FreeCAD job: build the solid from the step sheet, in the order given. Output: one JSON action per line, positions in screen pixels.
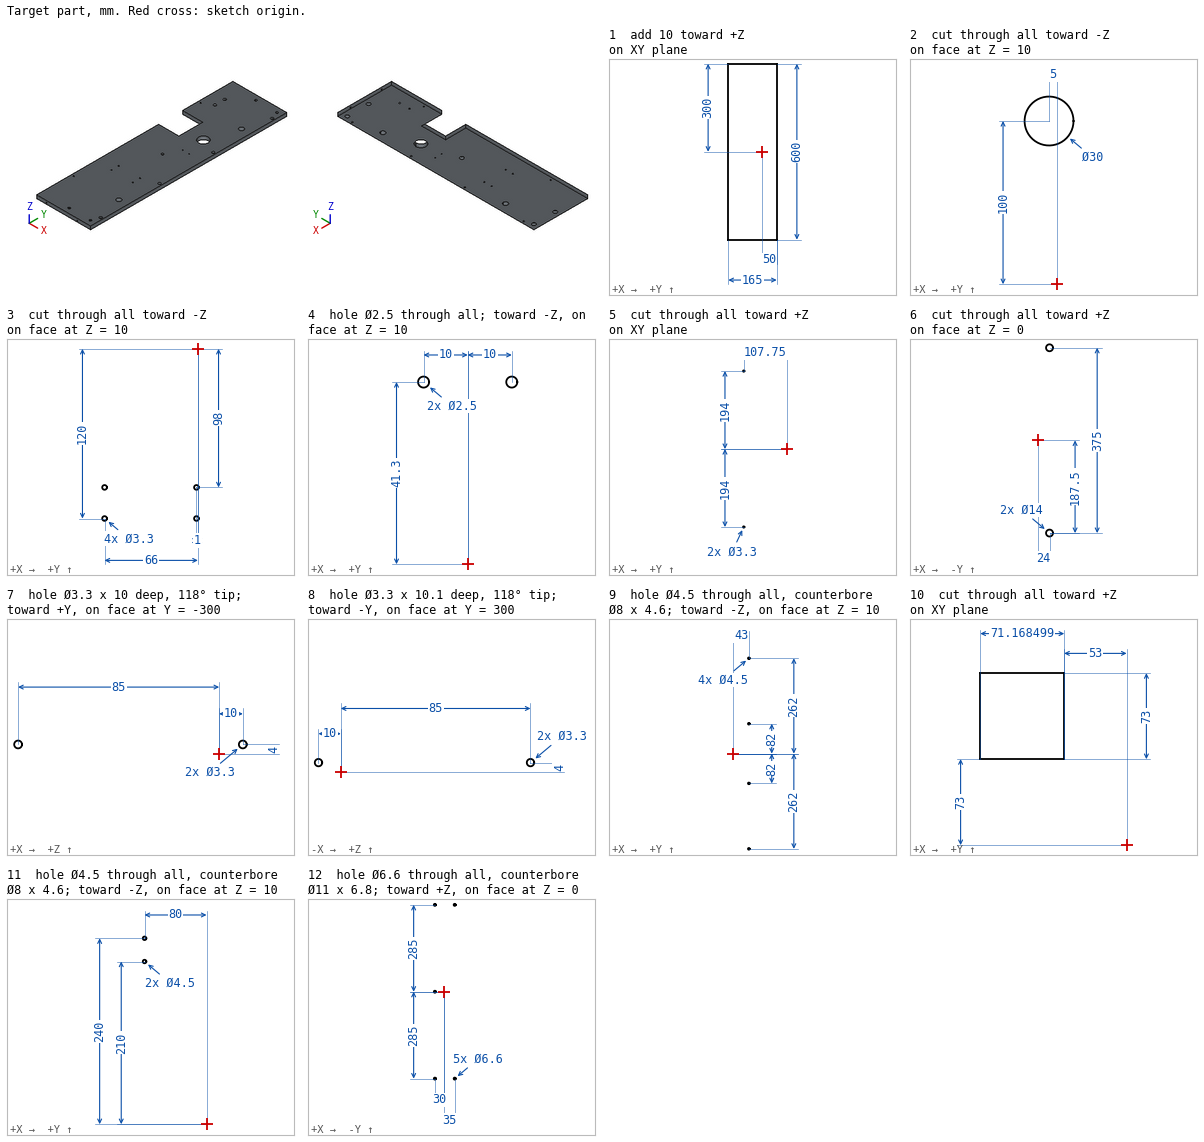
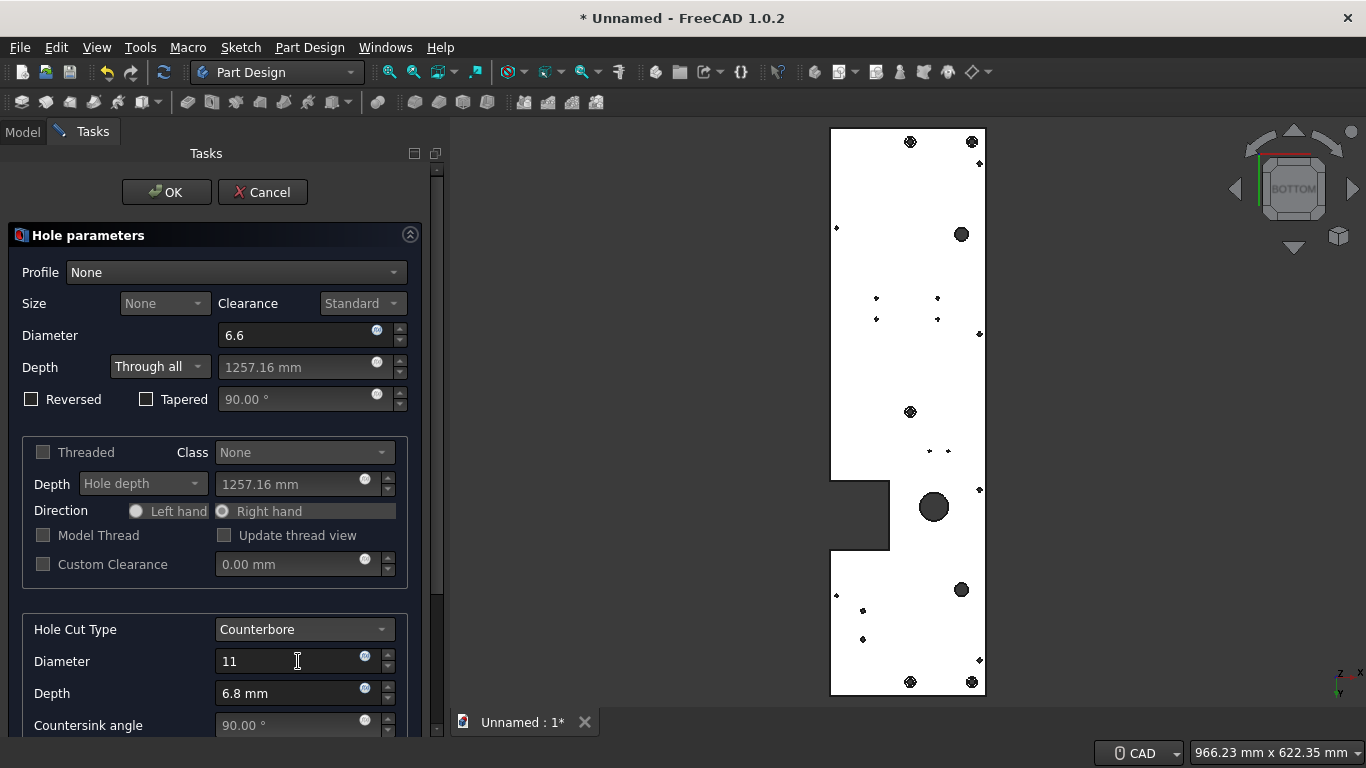
{"action": "left_click", "coordinate": [167, 192]}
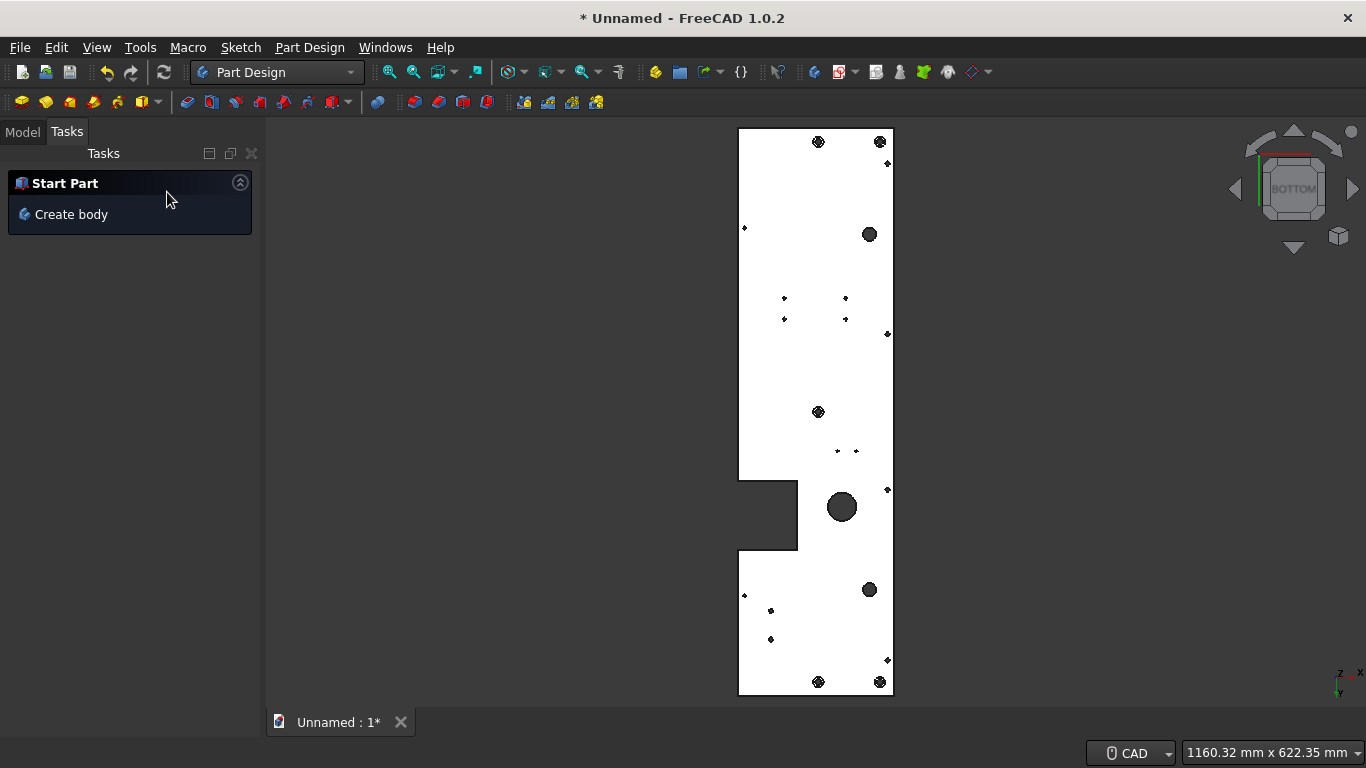
{"action": "key", "text": "0"}